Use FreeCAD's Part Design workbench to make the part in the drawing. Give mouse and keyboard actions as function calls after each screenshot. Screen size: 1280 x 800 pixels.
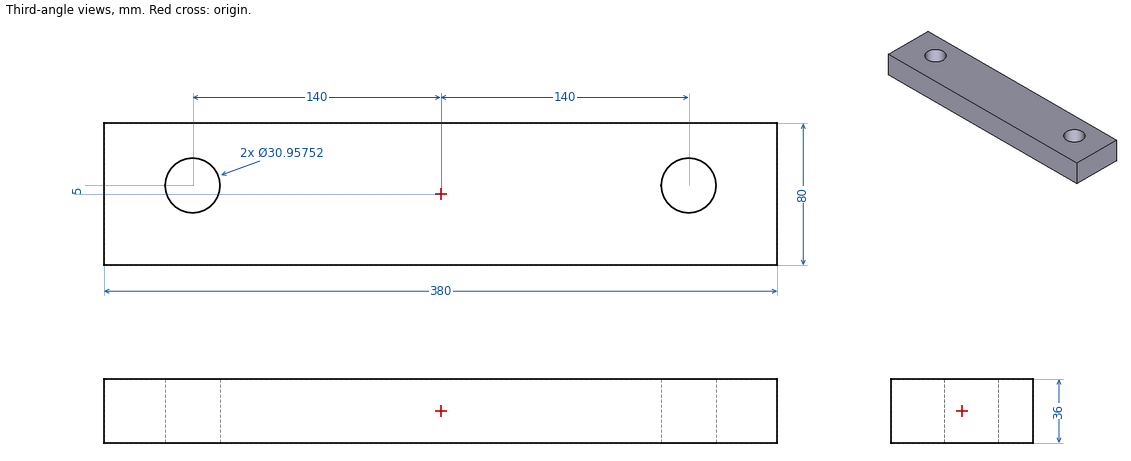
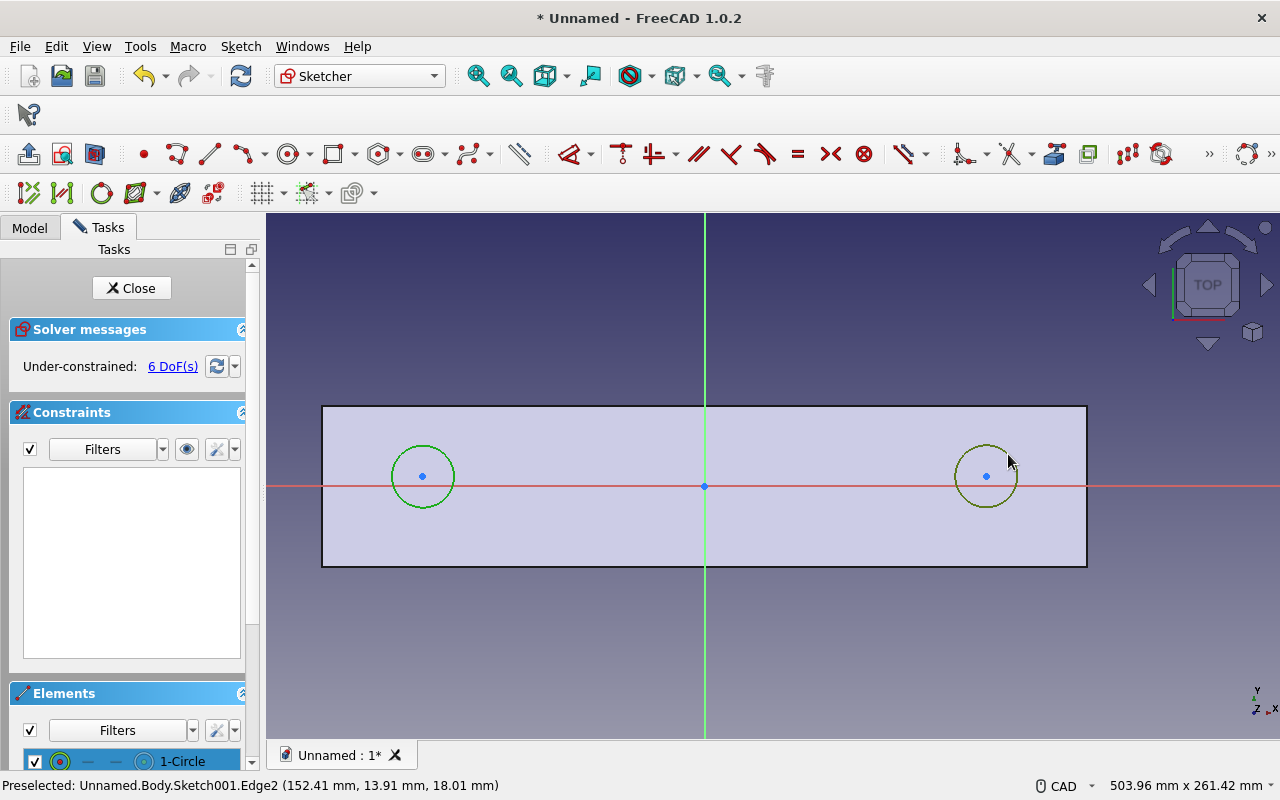
click(798, 154)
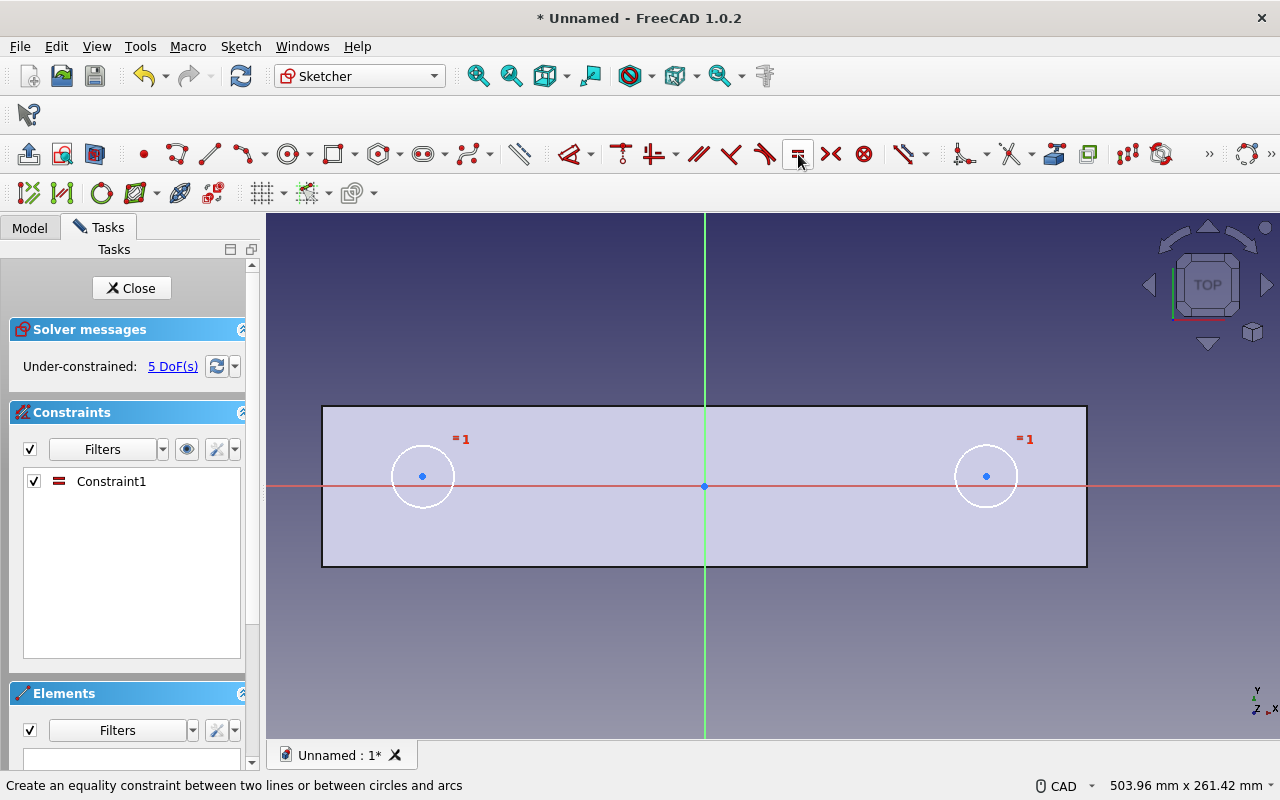
click(423, 477)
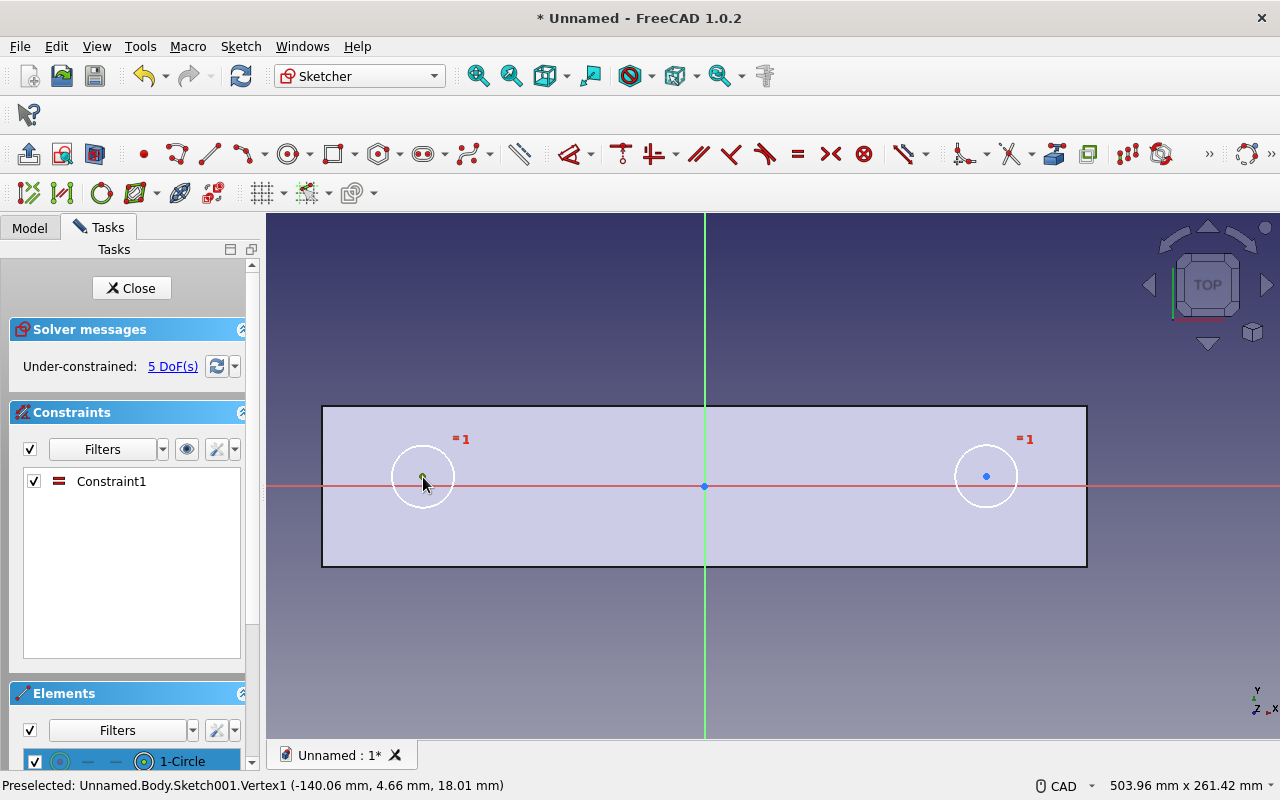
click(986, 476)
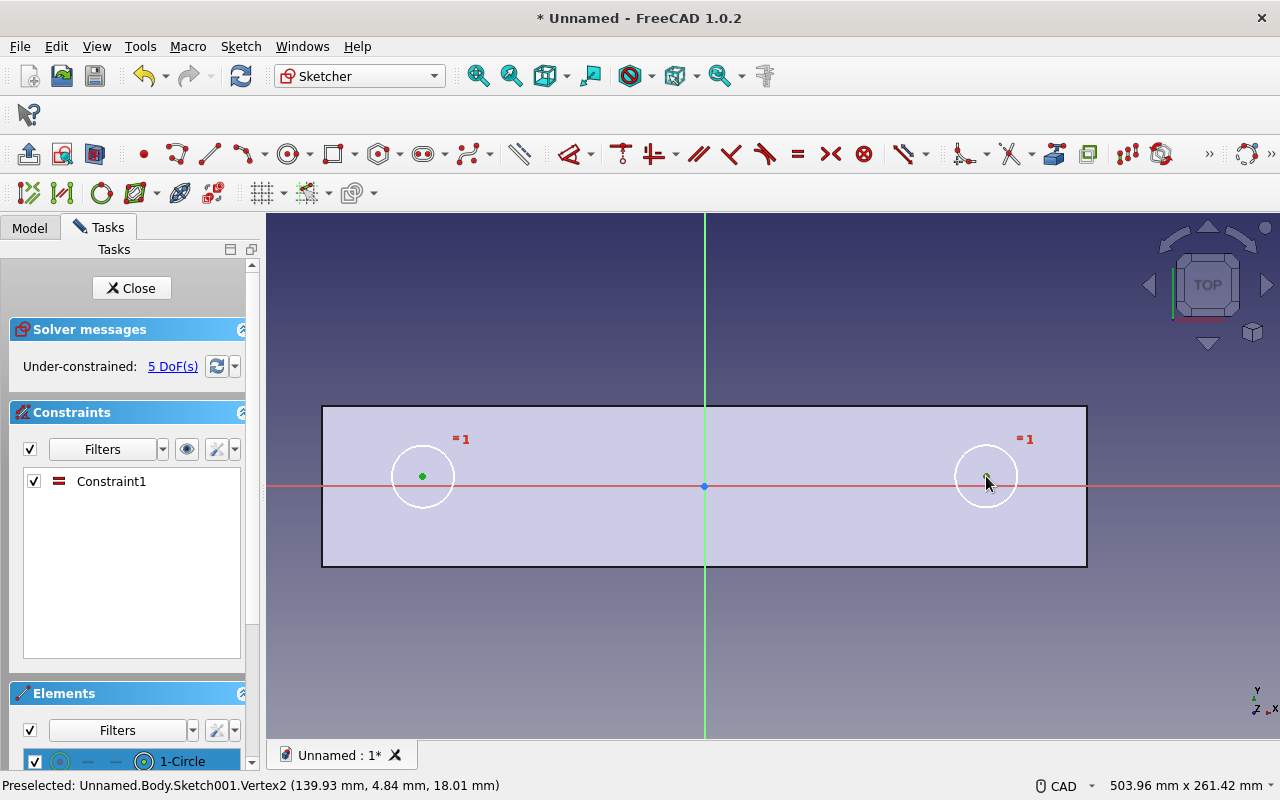
key(h)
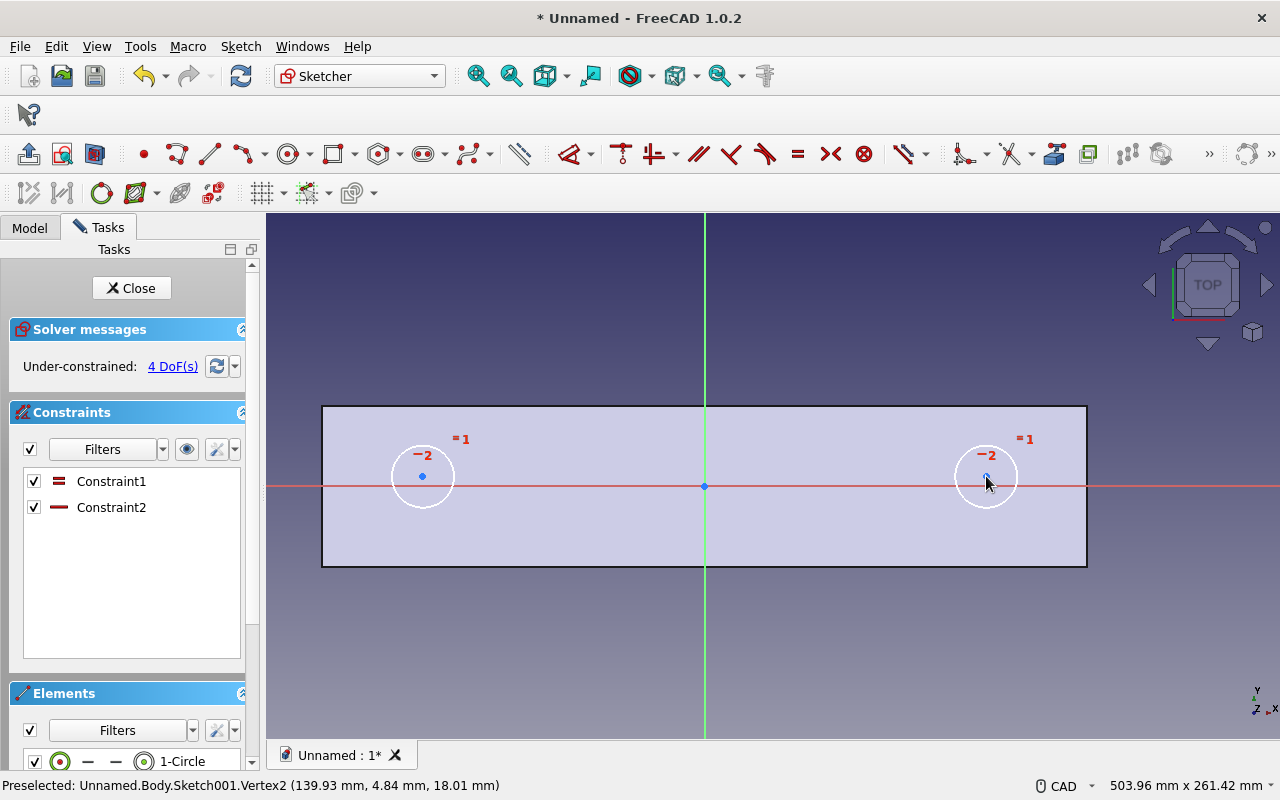
click(568, 154)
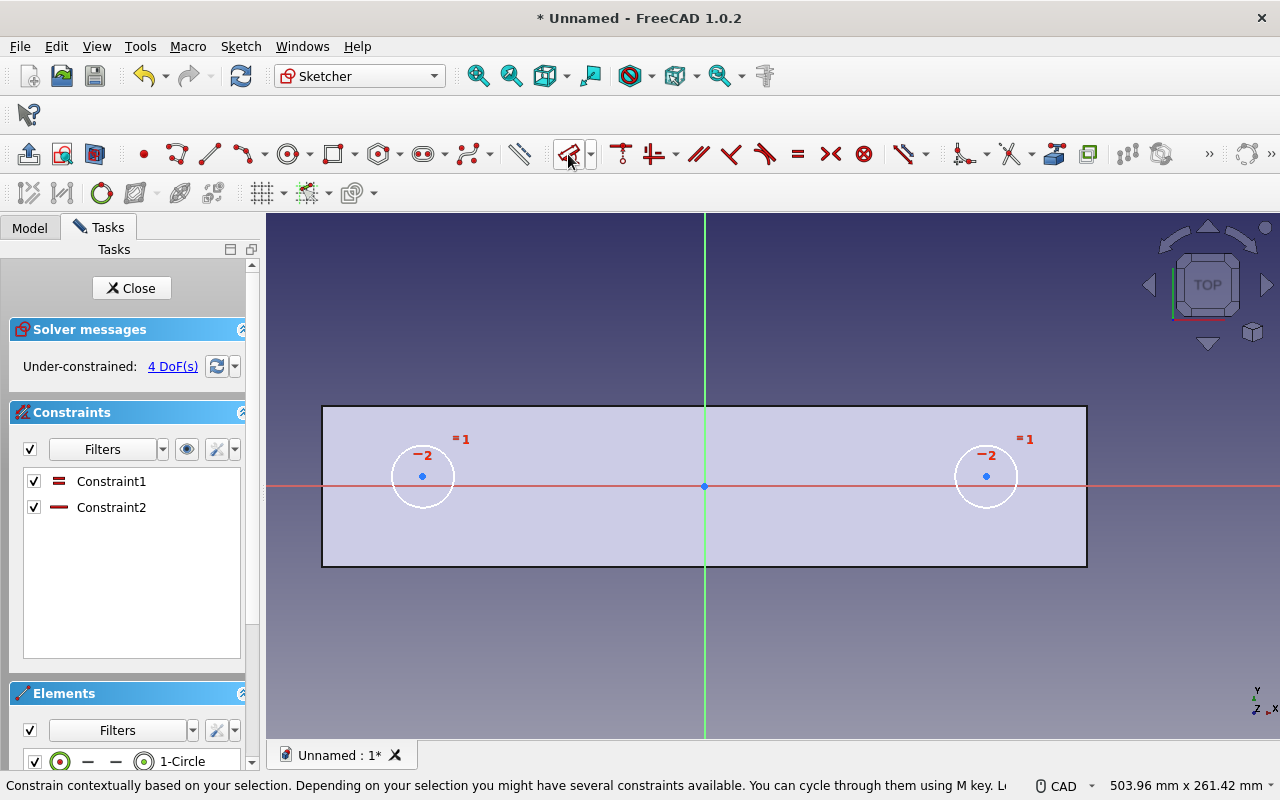
click(445, 455)
click(468, 433)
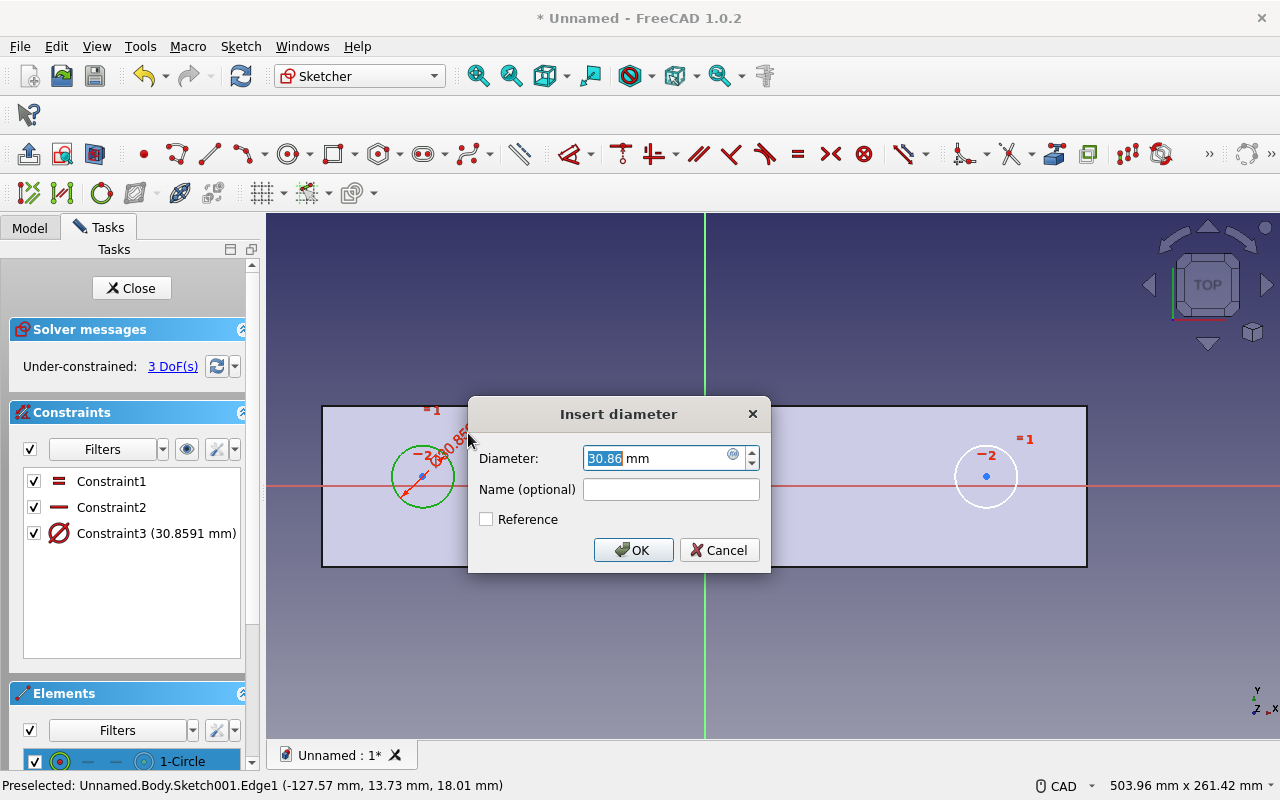
text(30.95752)
key(Return)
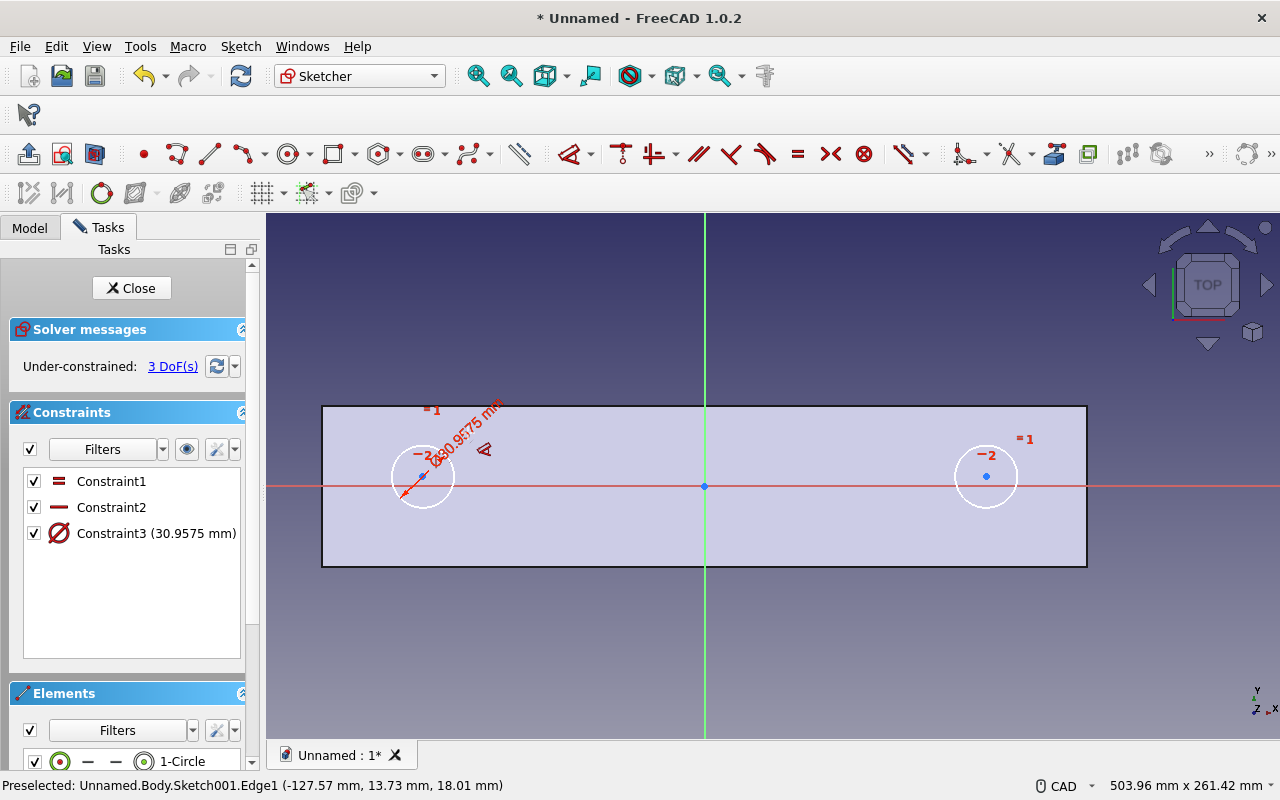
scroll(423, 477, up, 7)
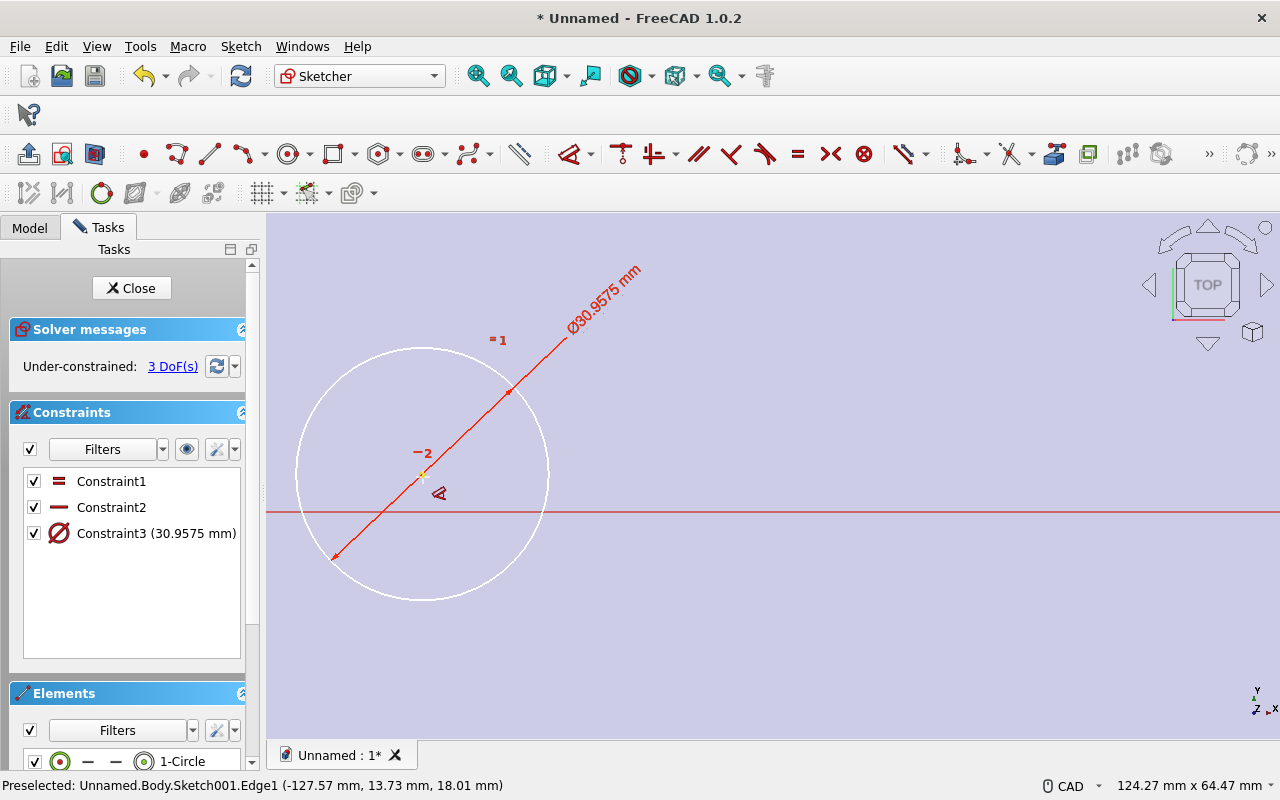
click(422, 474)
click(388, 493)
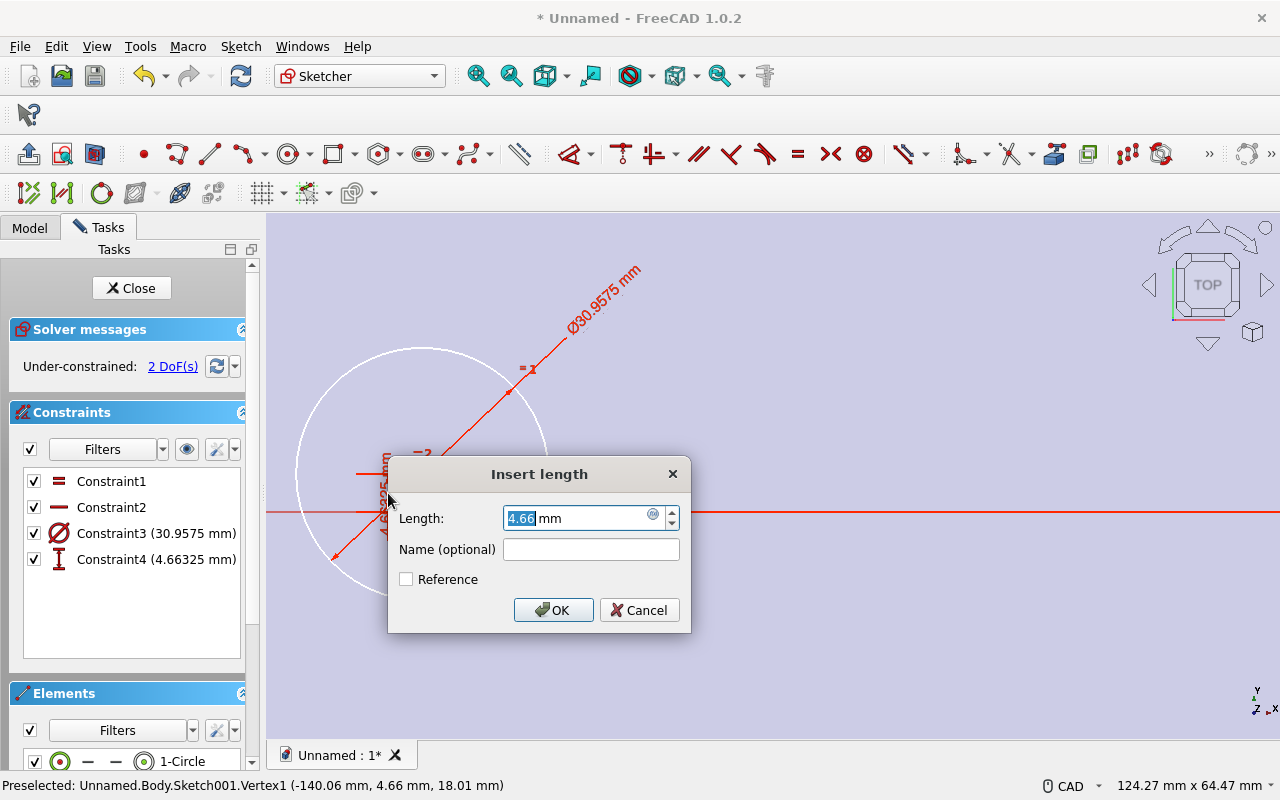
text(5)
key(Return)